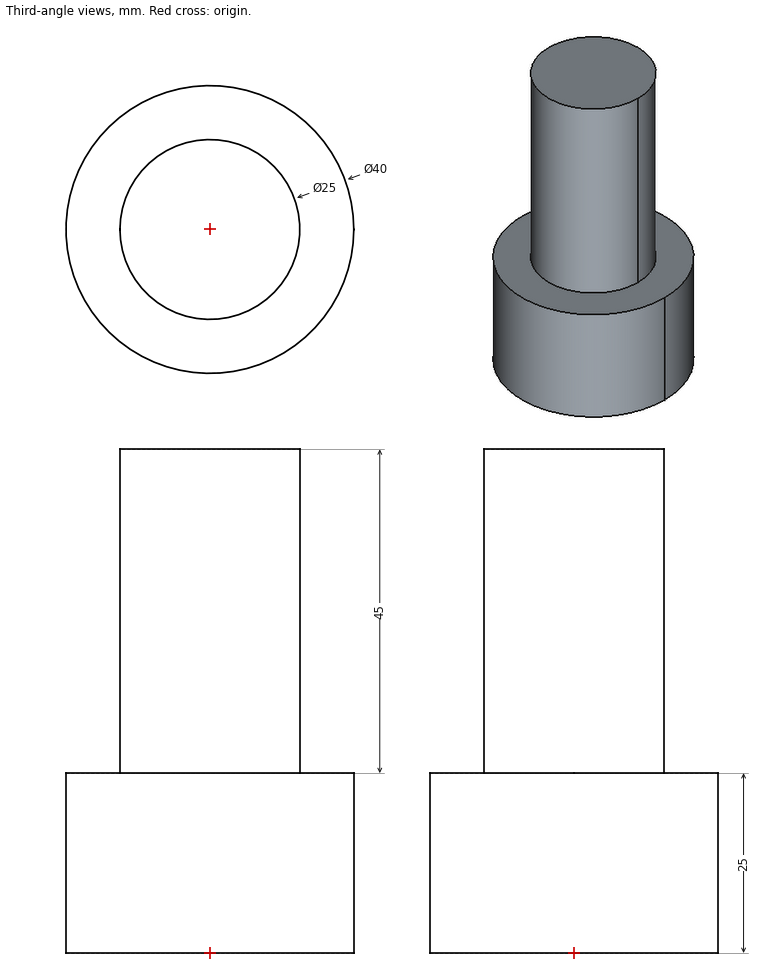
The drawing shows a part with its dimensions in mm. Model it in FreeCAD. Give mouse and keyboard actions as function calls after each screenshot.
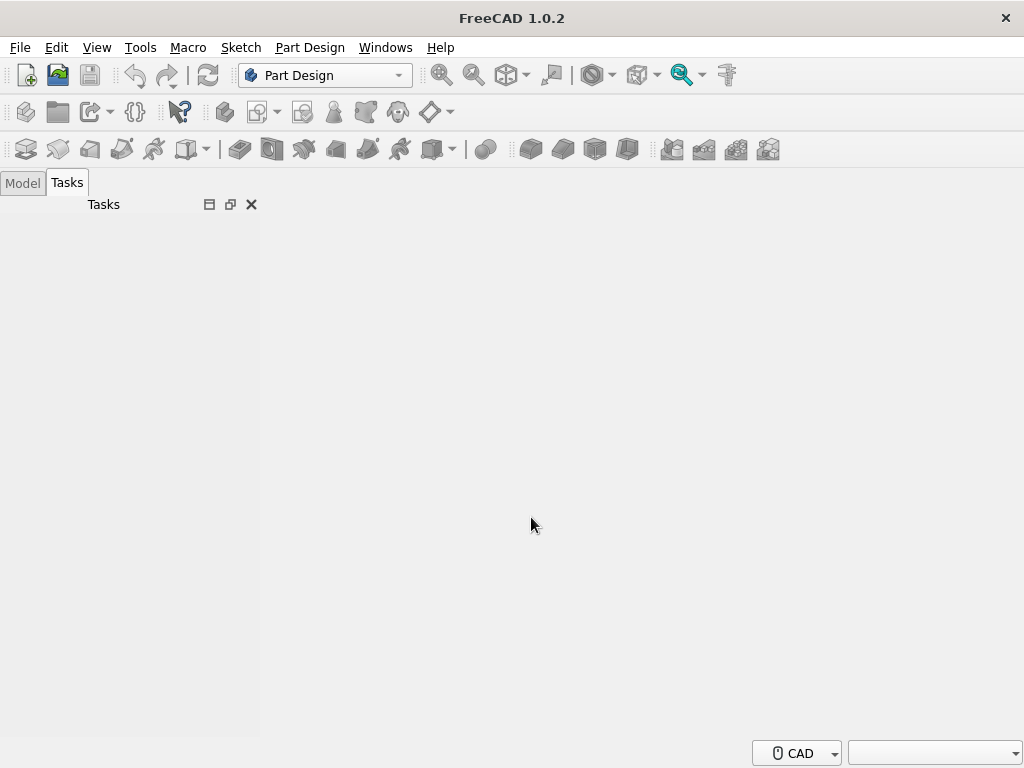
click(26, 76)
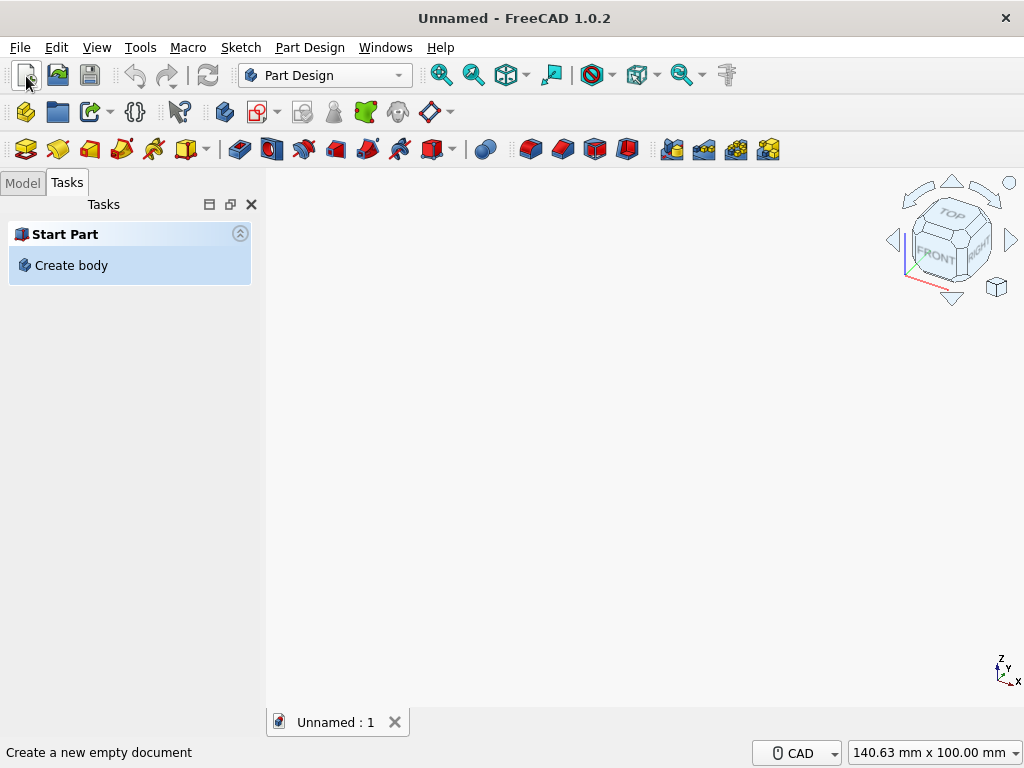
click(258, 112)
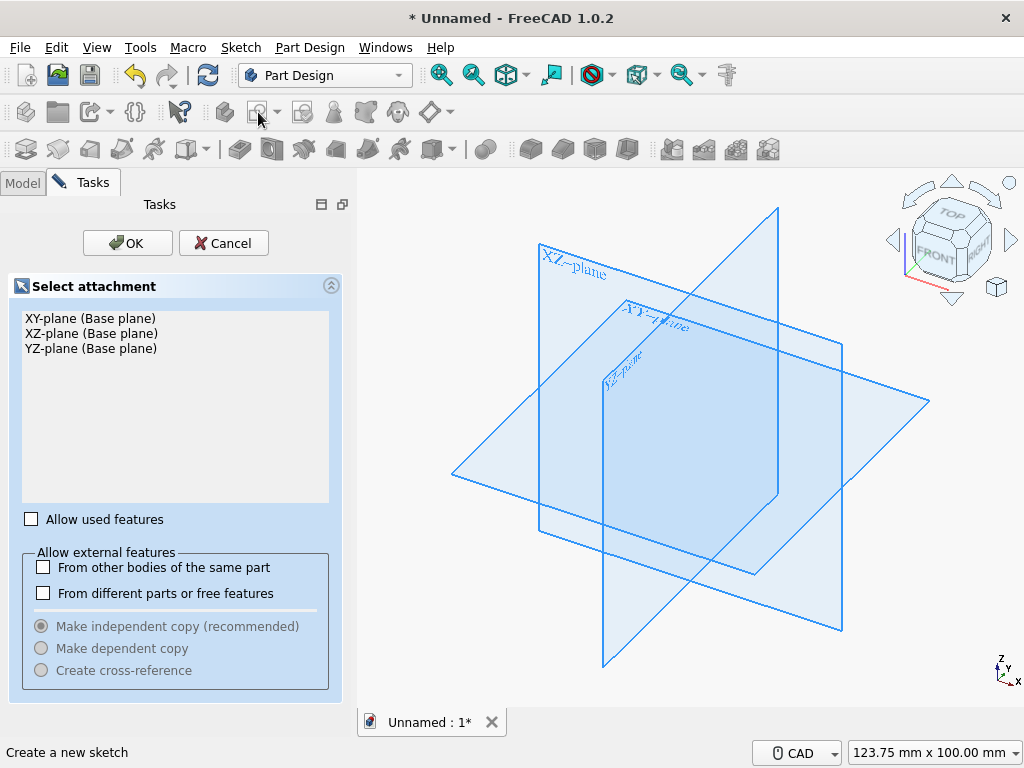
click(82, 318)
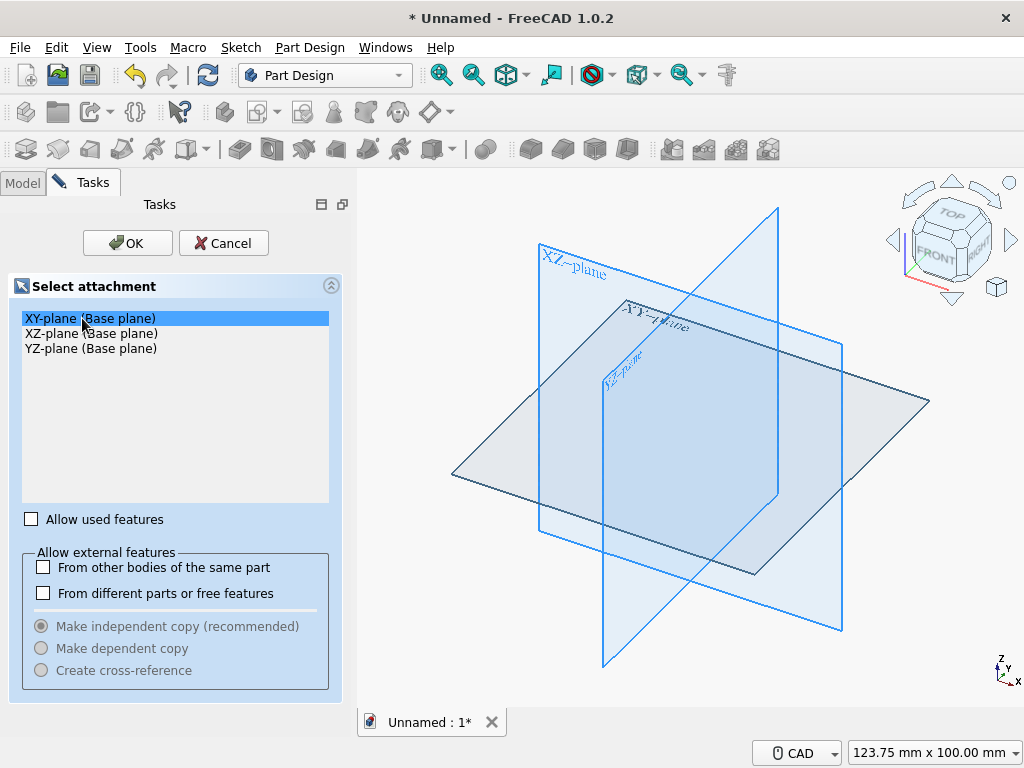
click(128, 243)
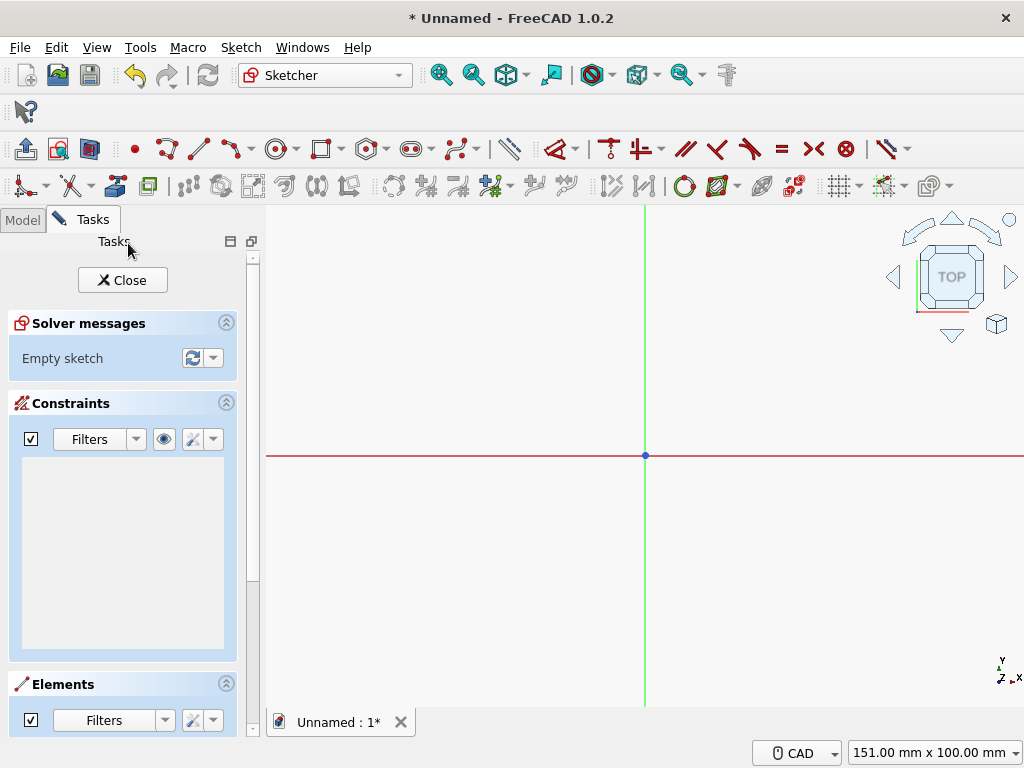
scroll(784, 456, up, 2)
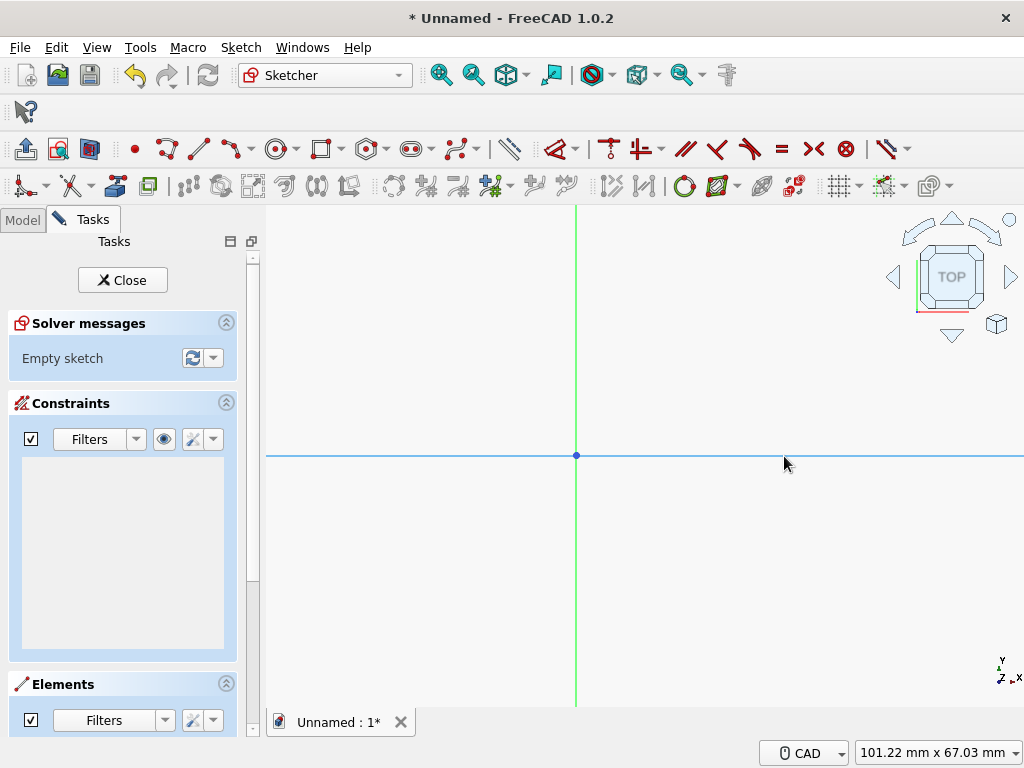
click(276, 150)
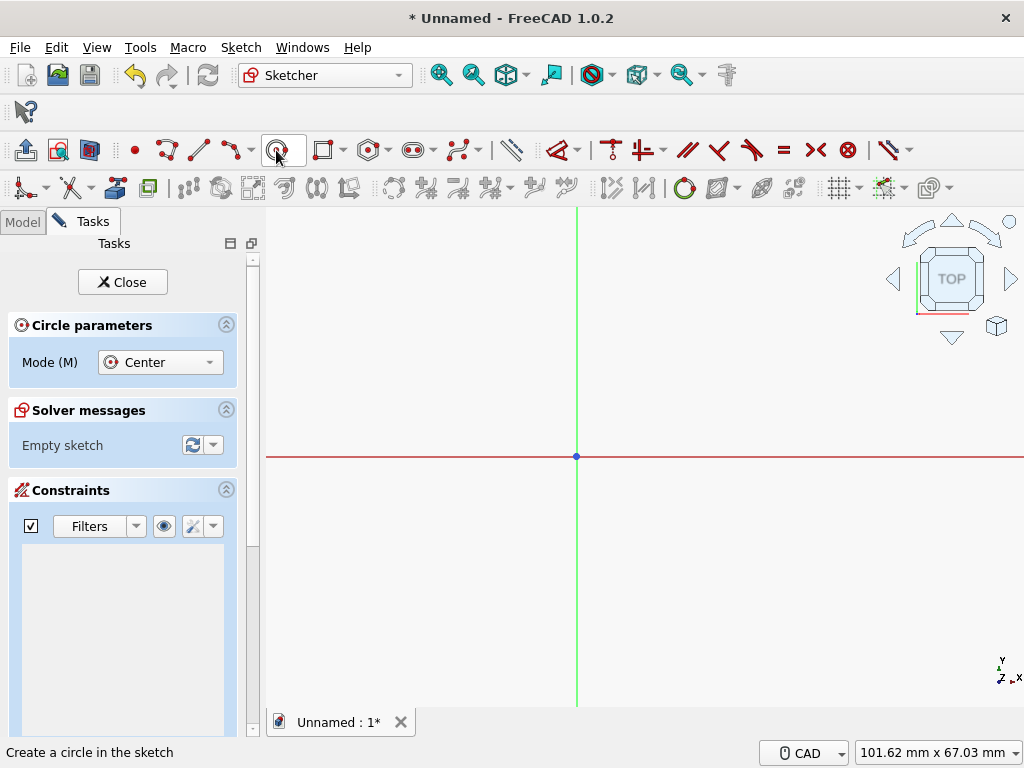
click(577, 457)
click(682, 351)
key(Escape)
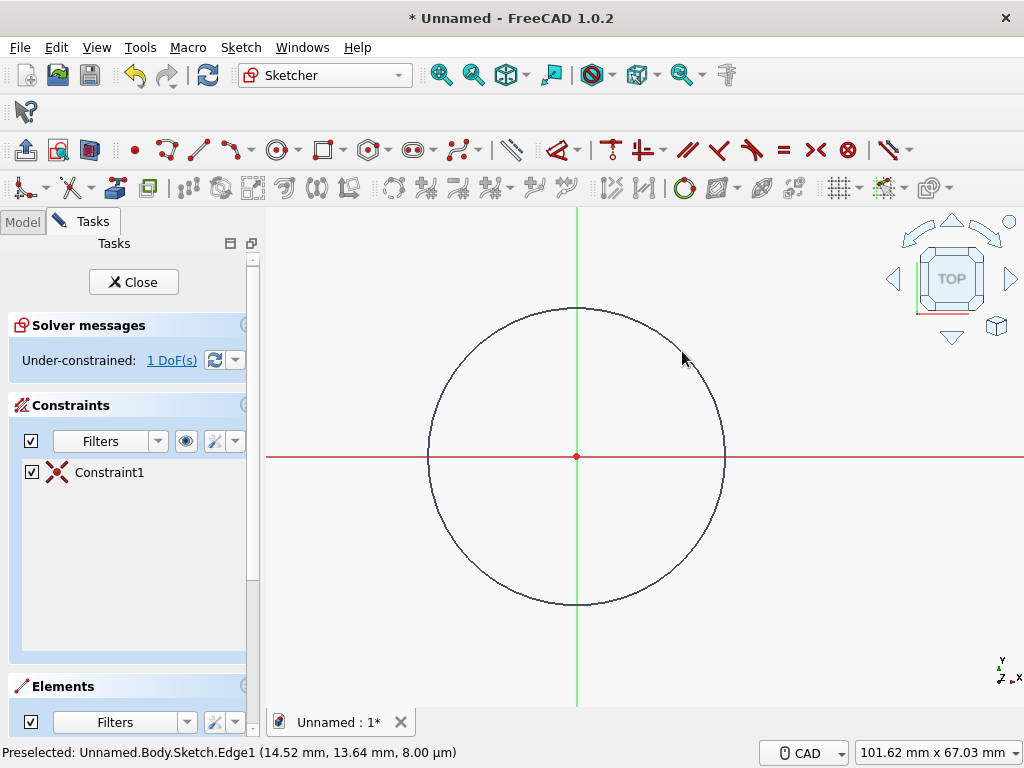
click(681, 351)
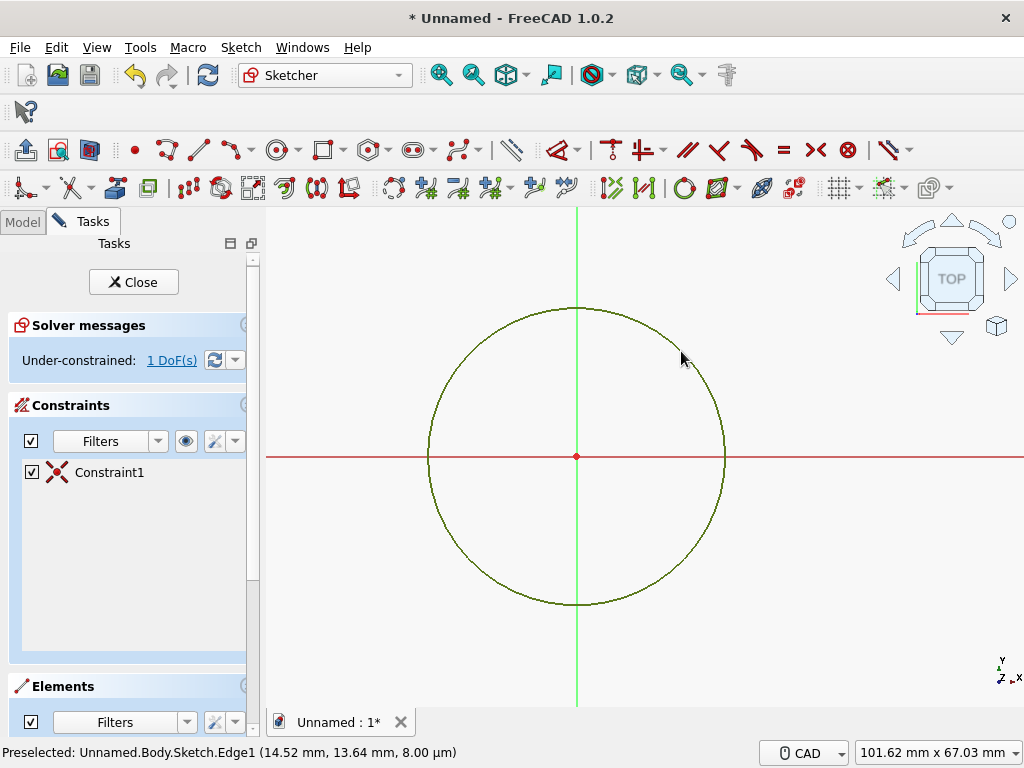
key(k)
key(o)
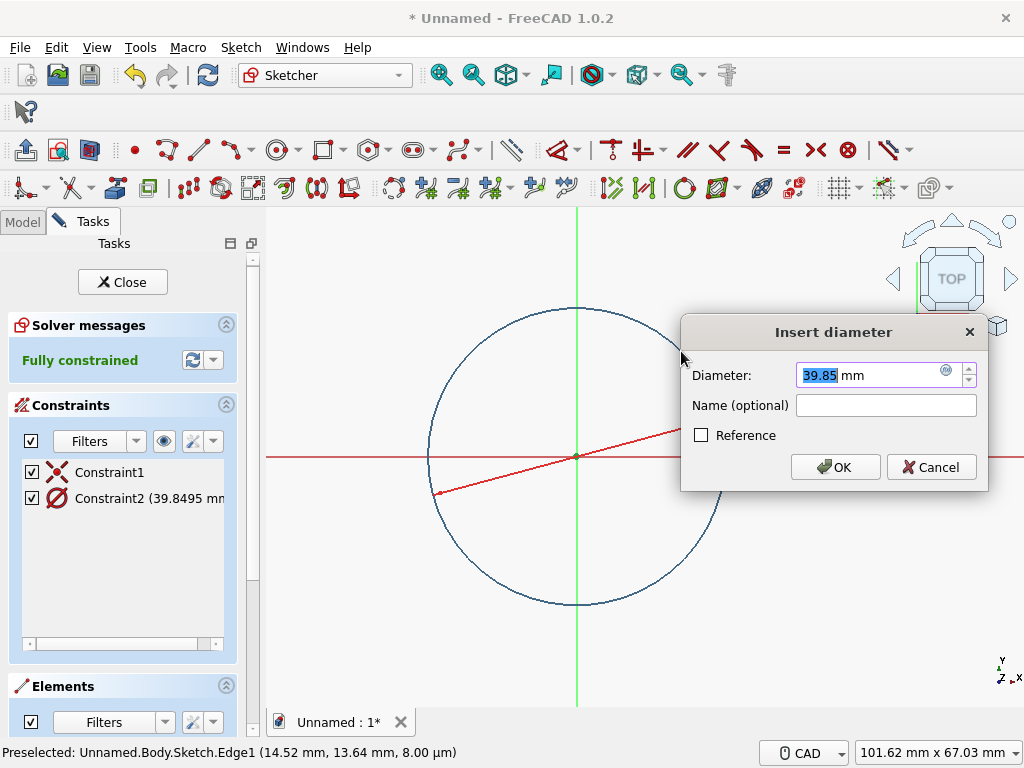
text(40)
key(Return)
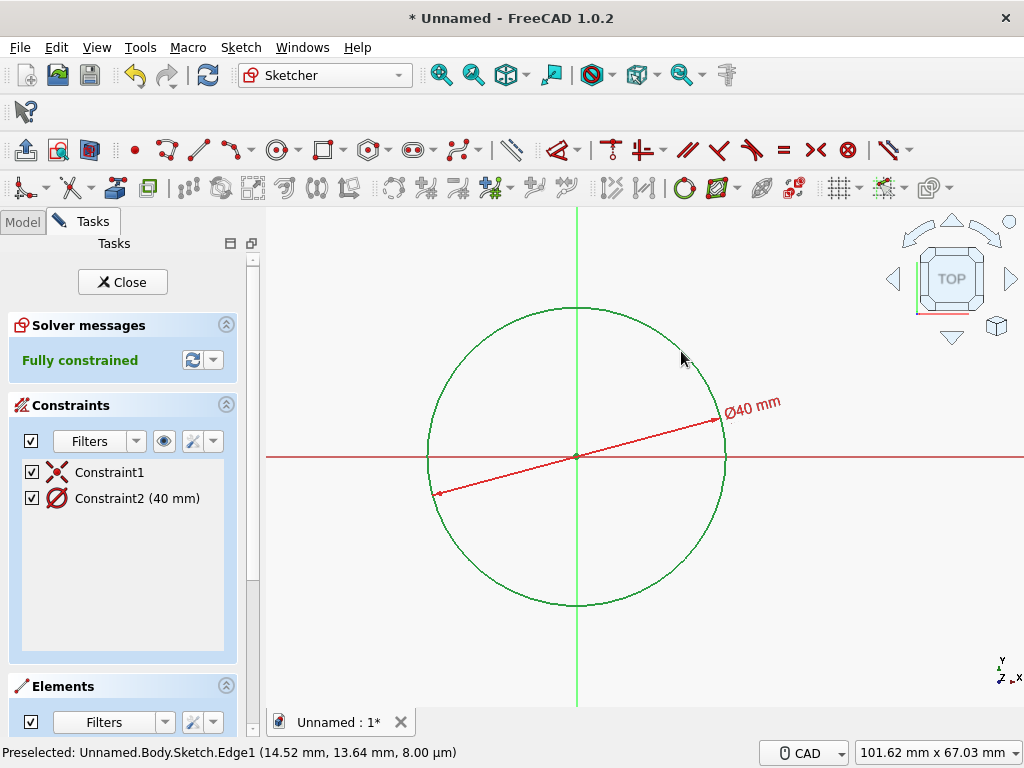
click(123, 282)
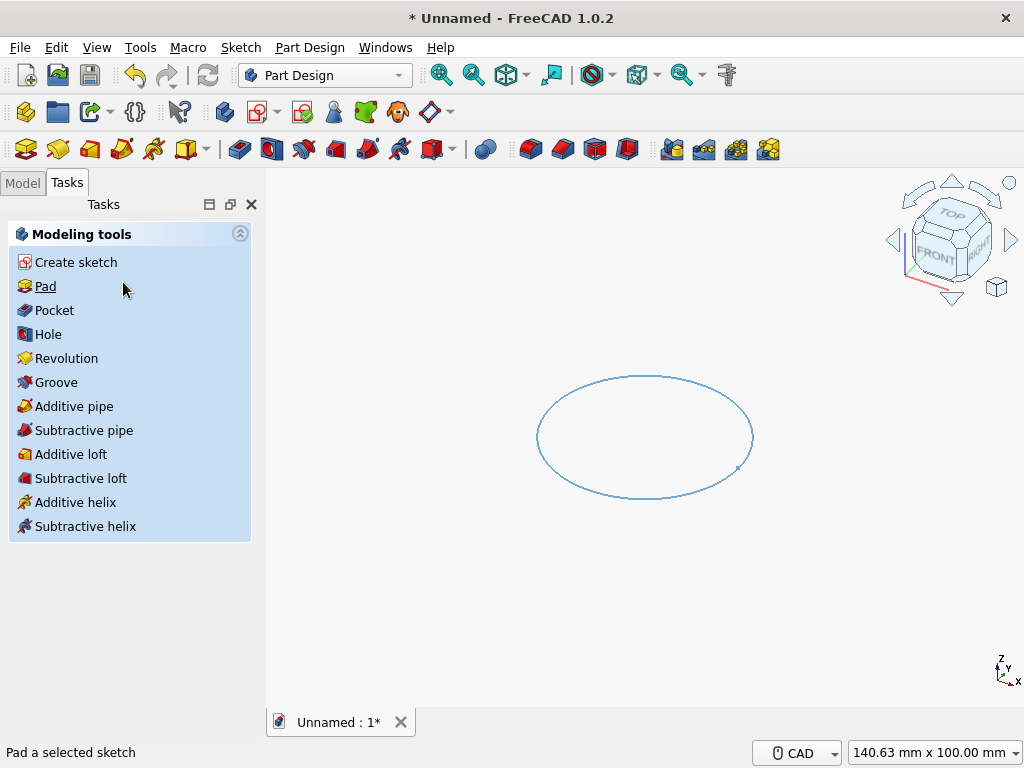
click(26, 150)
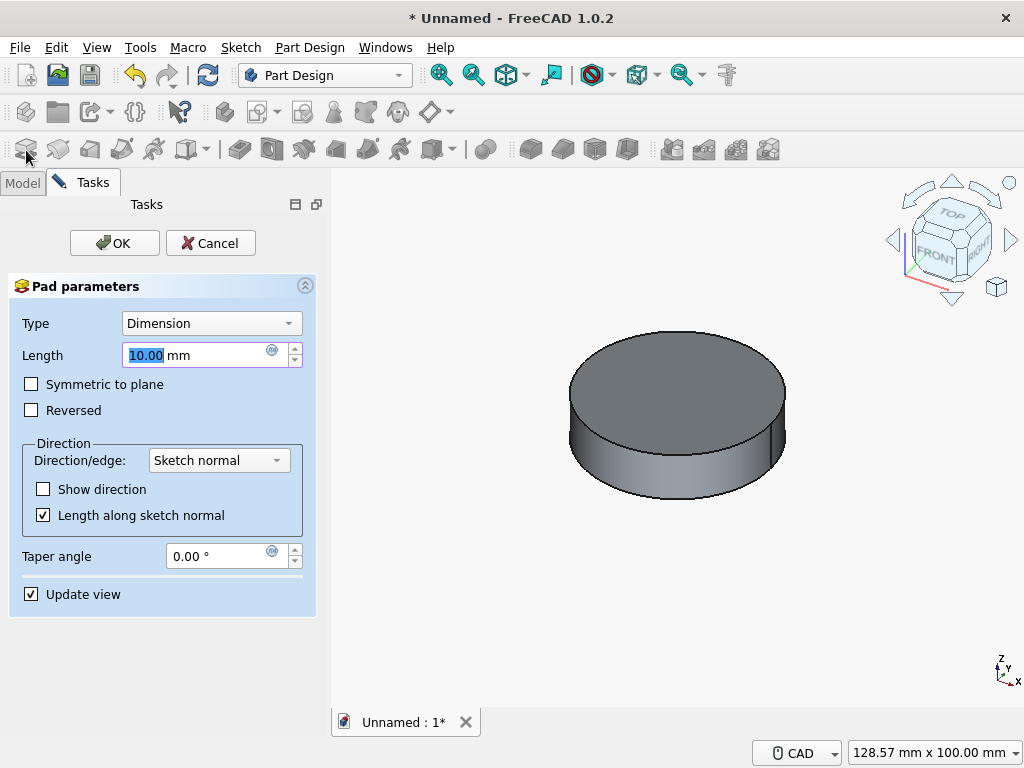
text(25)
key(Tab)